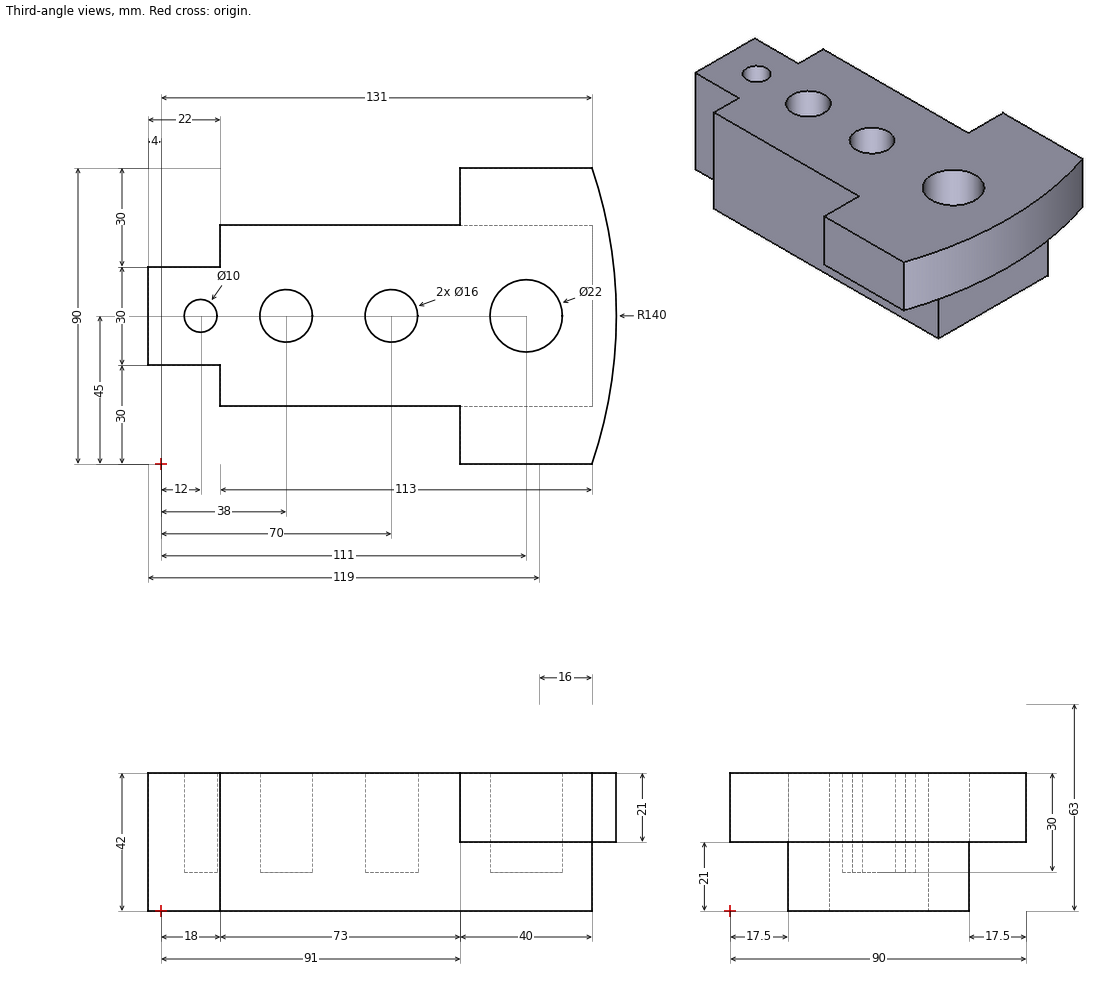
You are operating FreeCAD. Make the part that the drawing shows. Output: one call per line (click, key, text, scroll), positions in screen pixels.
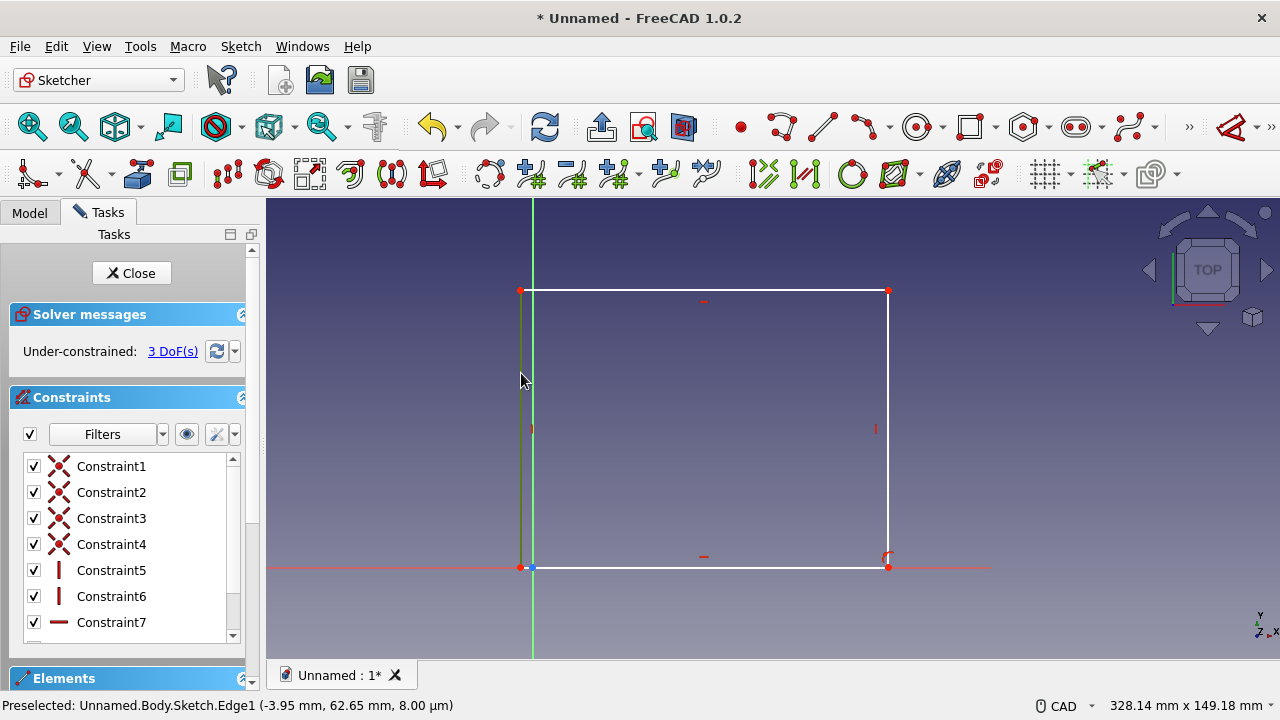
click(1256, 128)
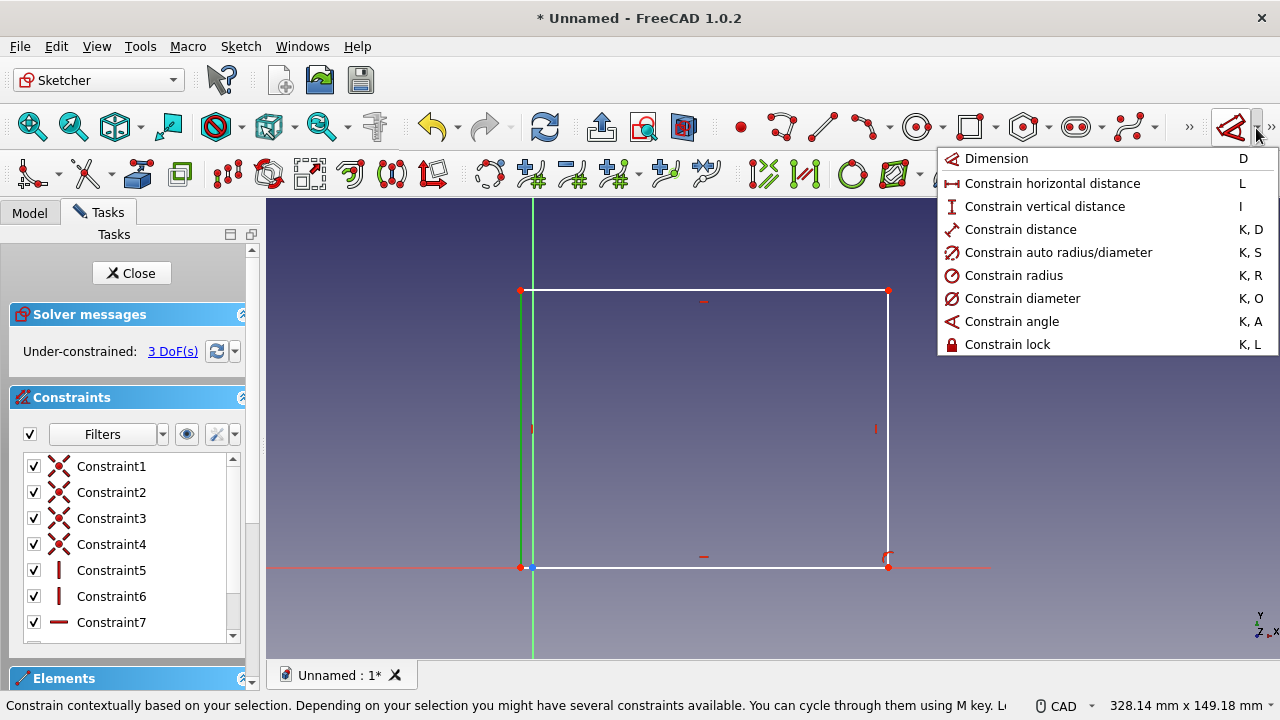
click(1108, 206)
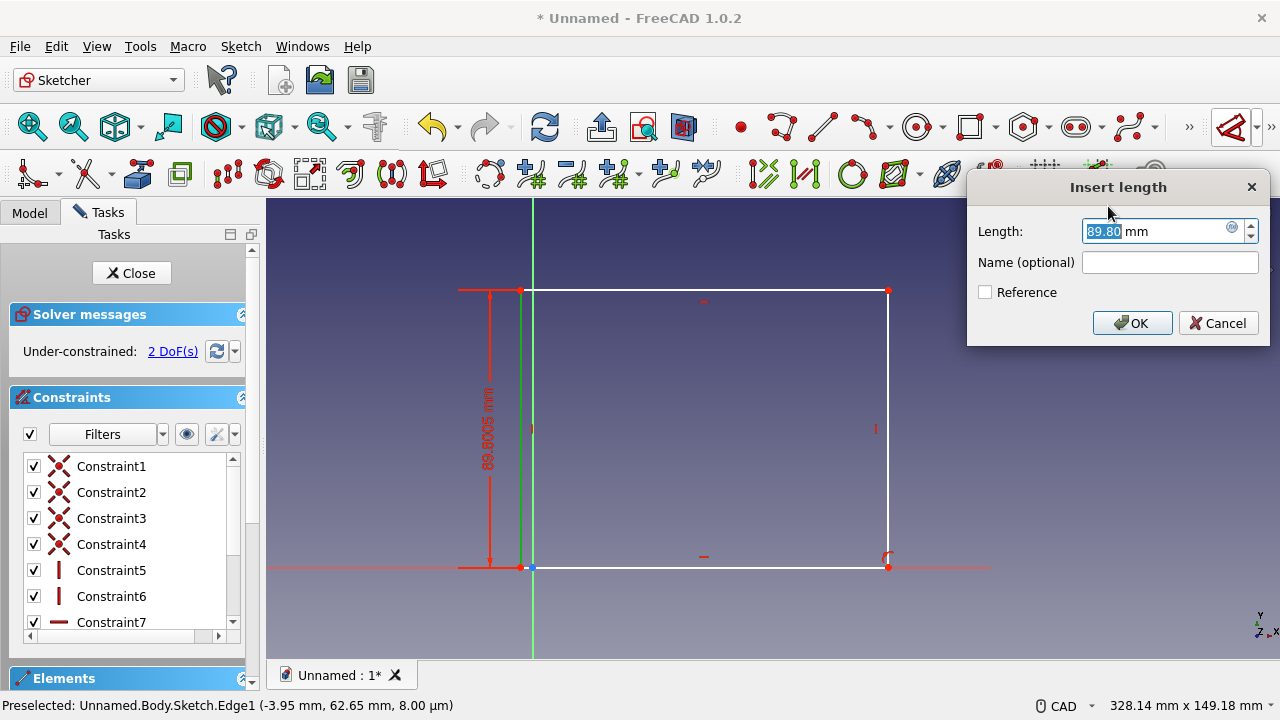
text(90)
key(Return)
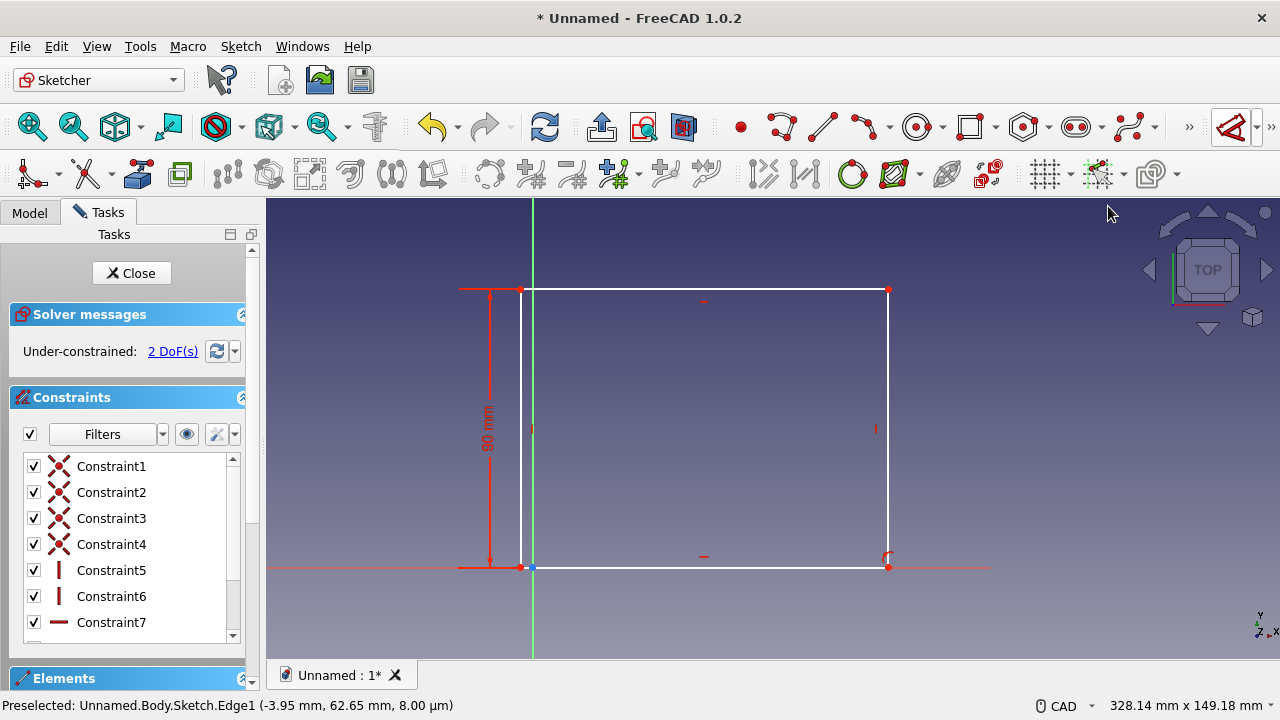
scroll(521, 289, up, 6)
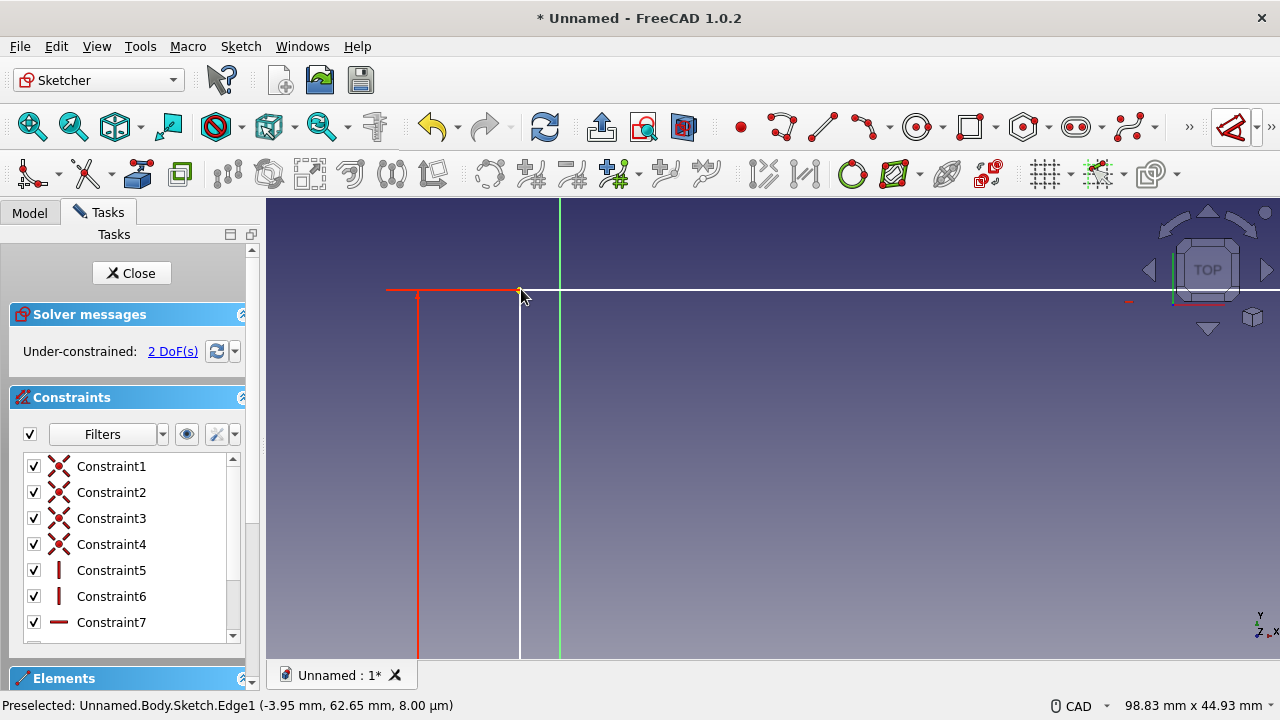
click(520, 290)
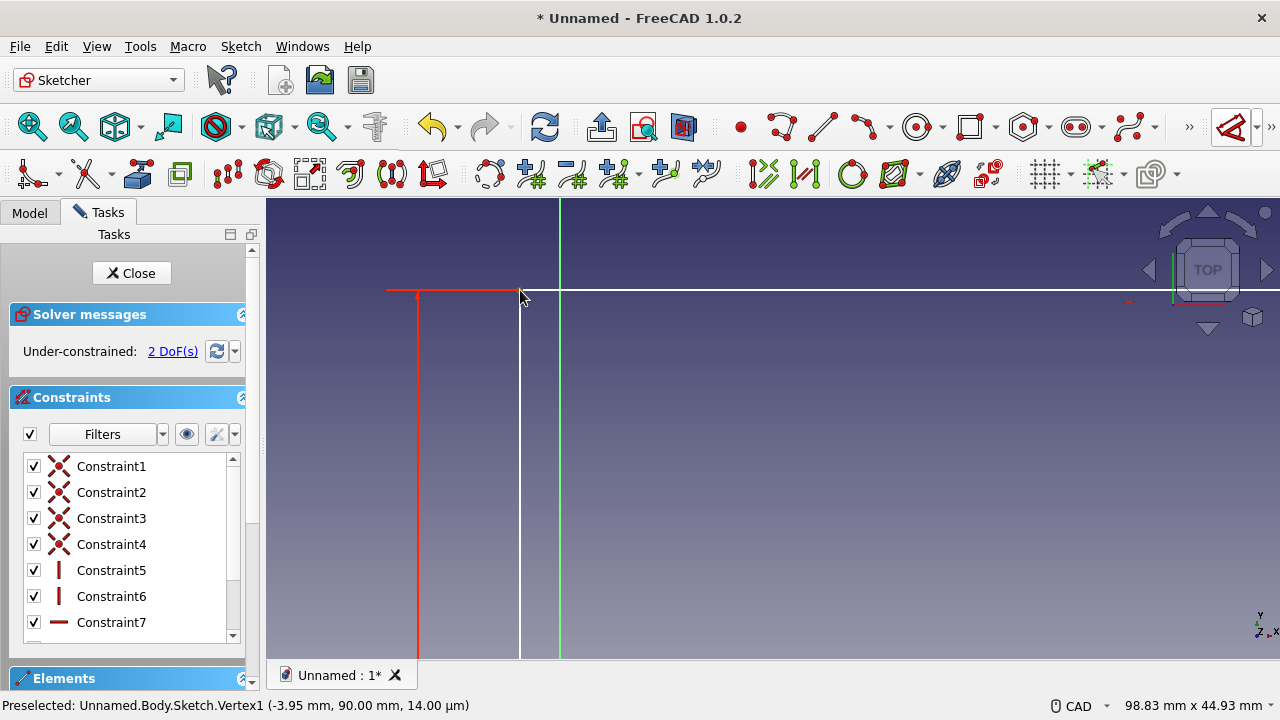
key(l)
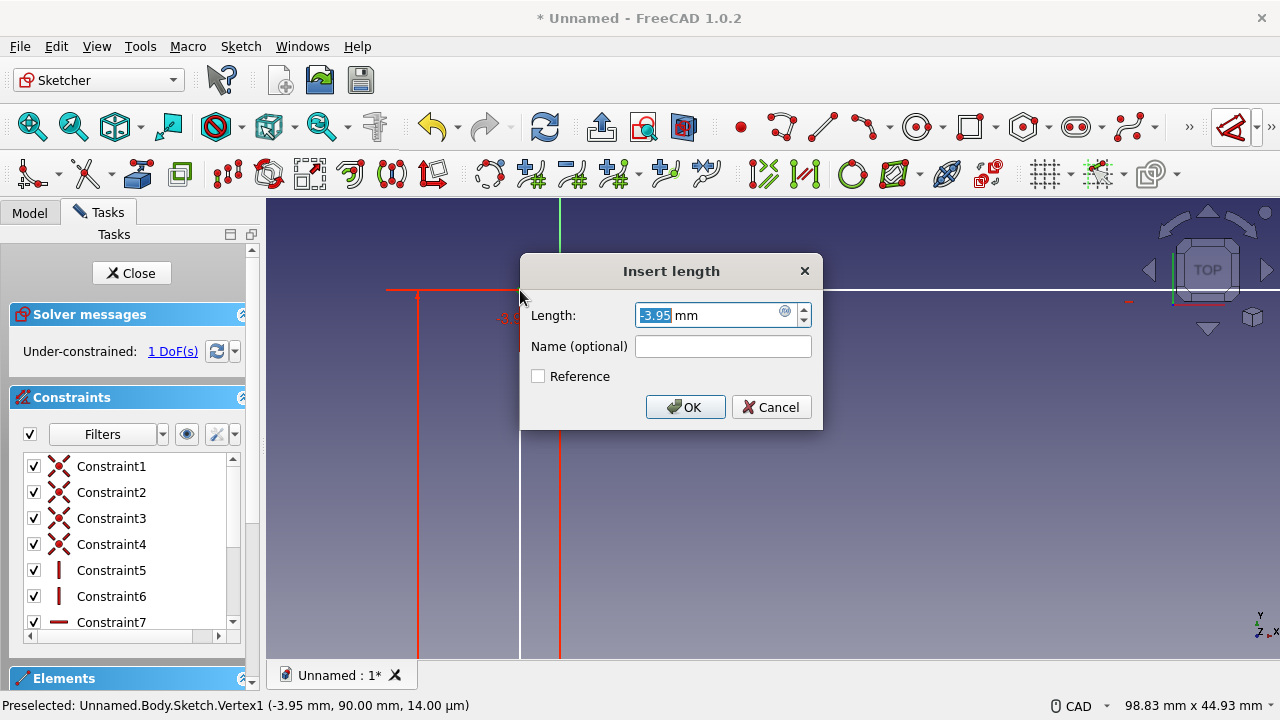
text(-4)
key(Return)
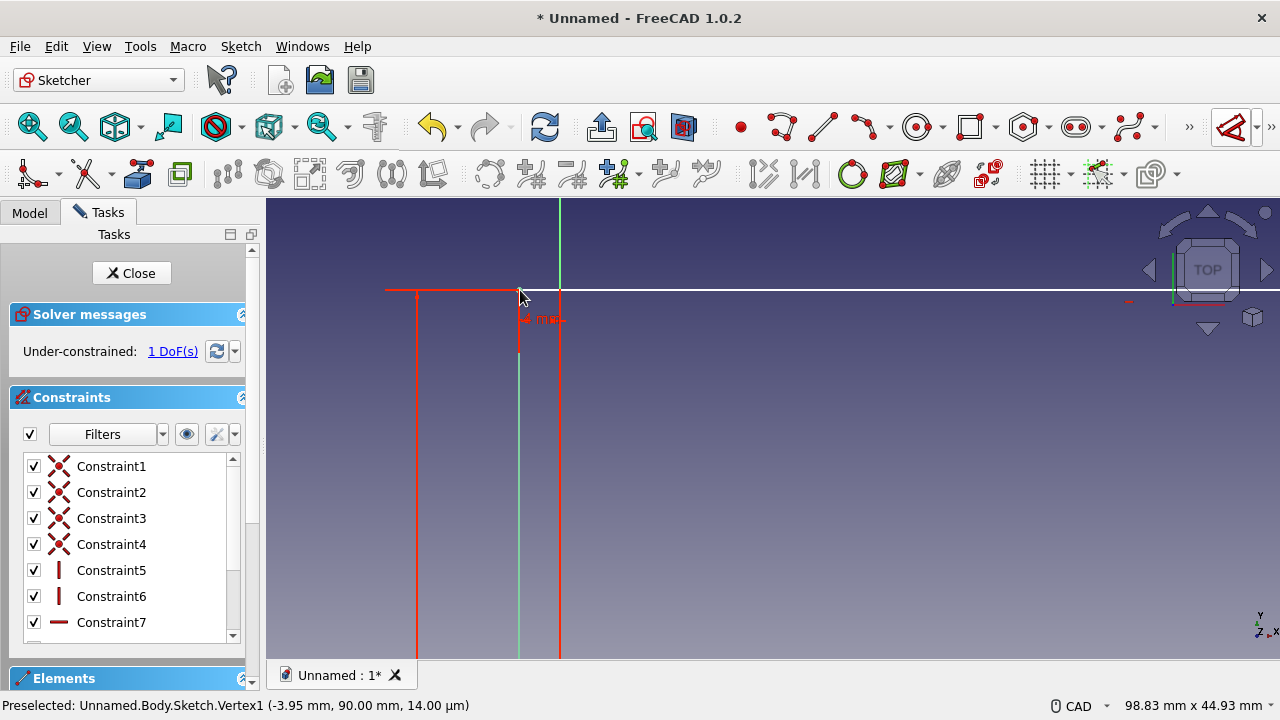
scroll(521, 289, down, 6)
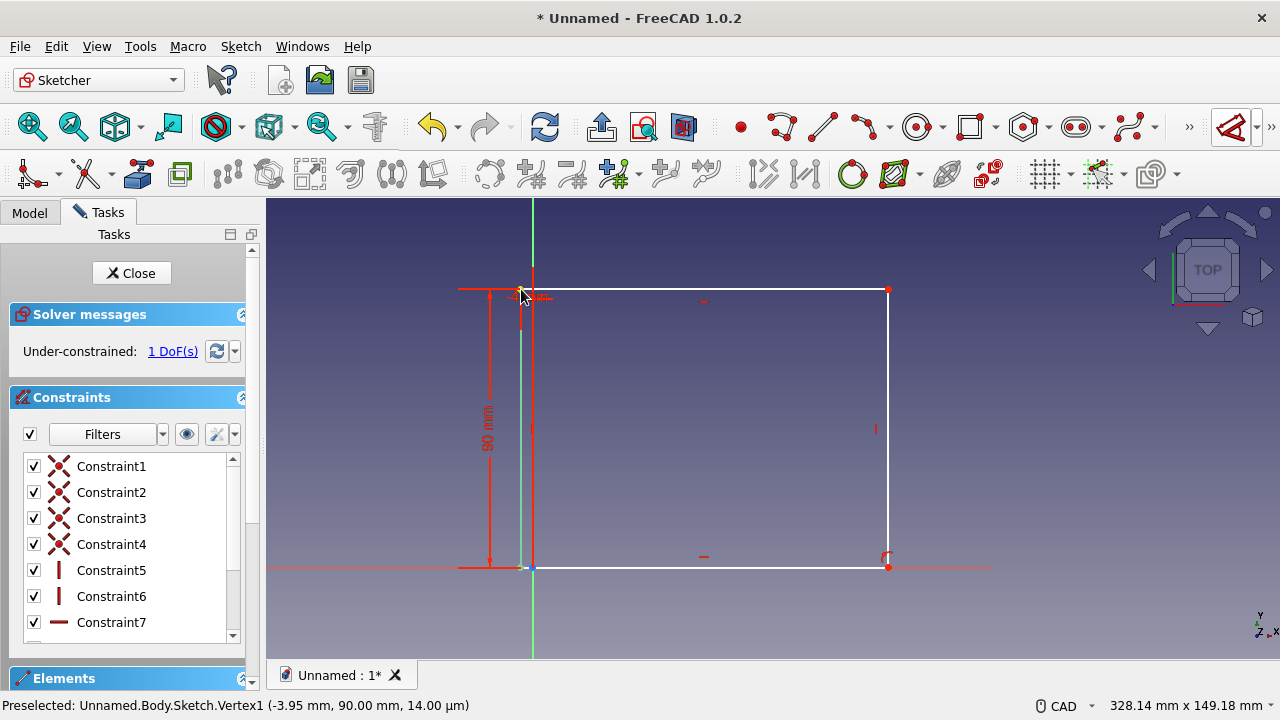
click(631, 568)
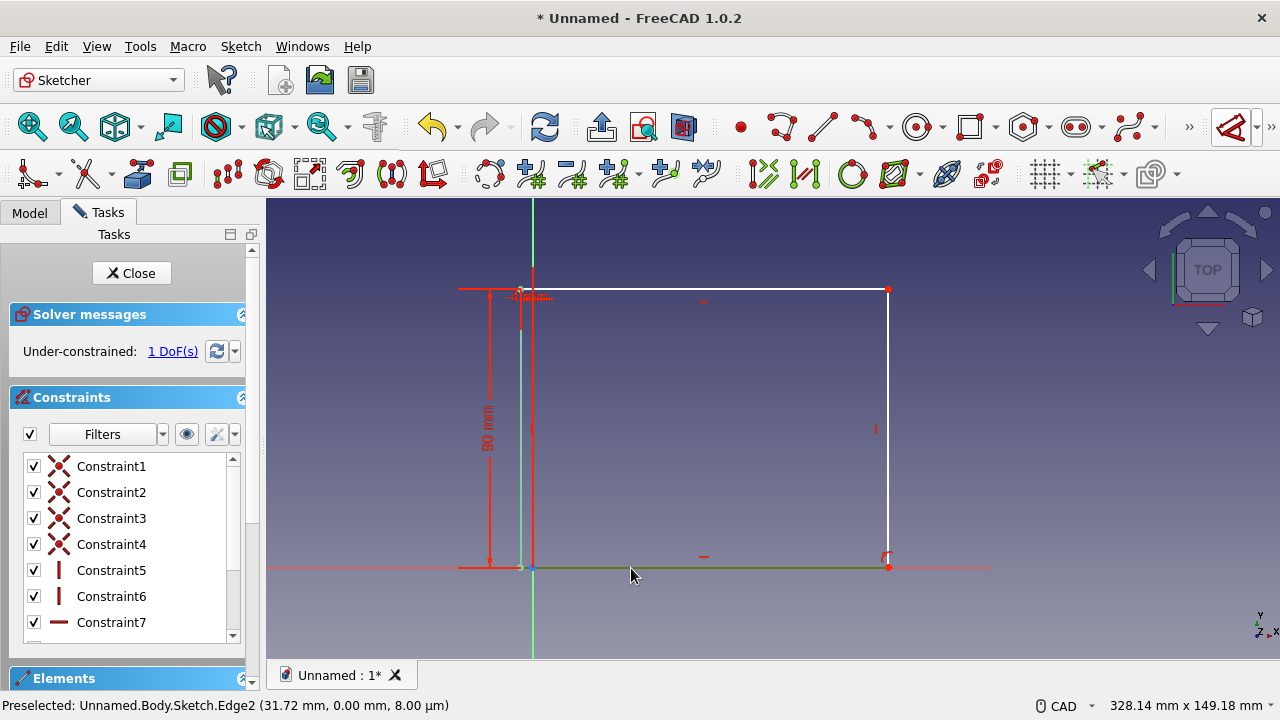
key(l)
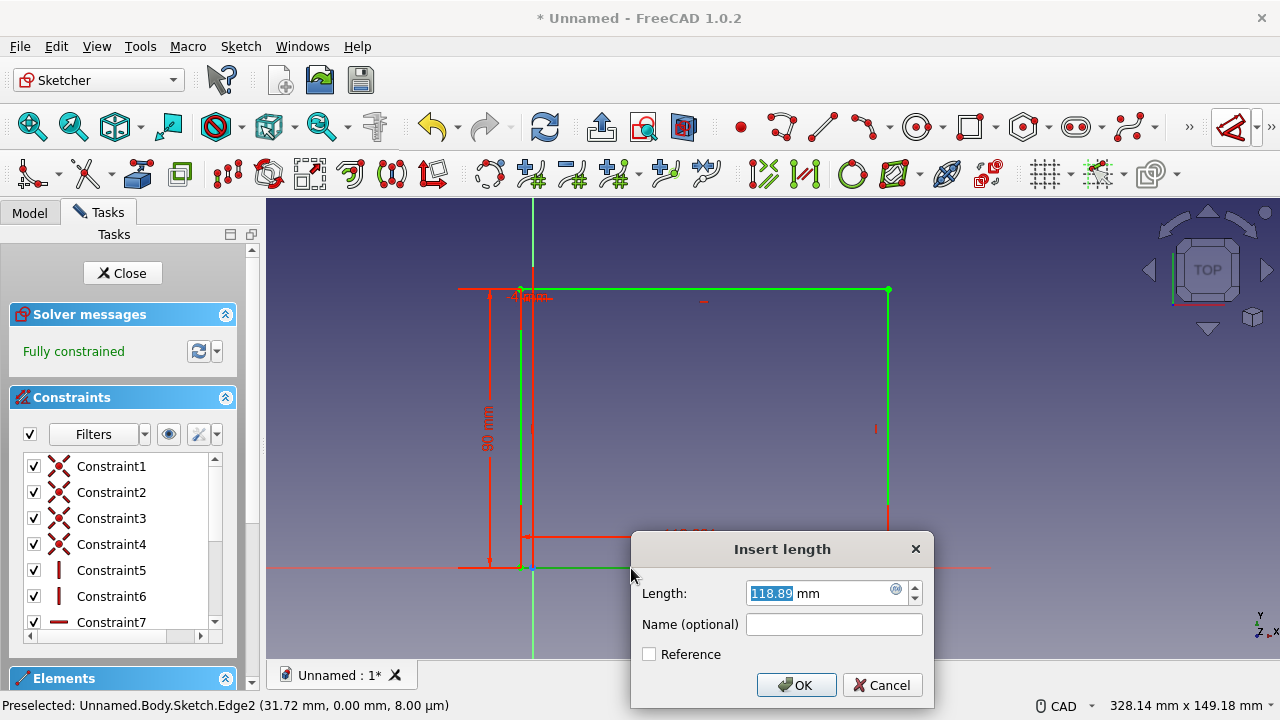
text(119)
key(Return)